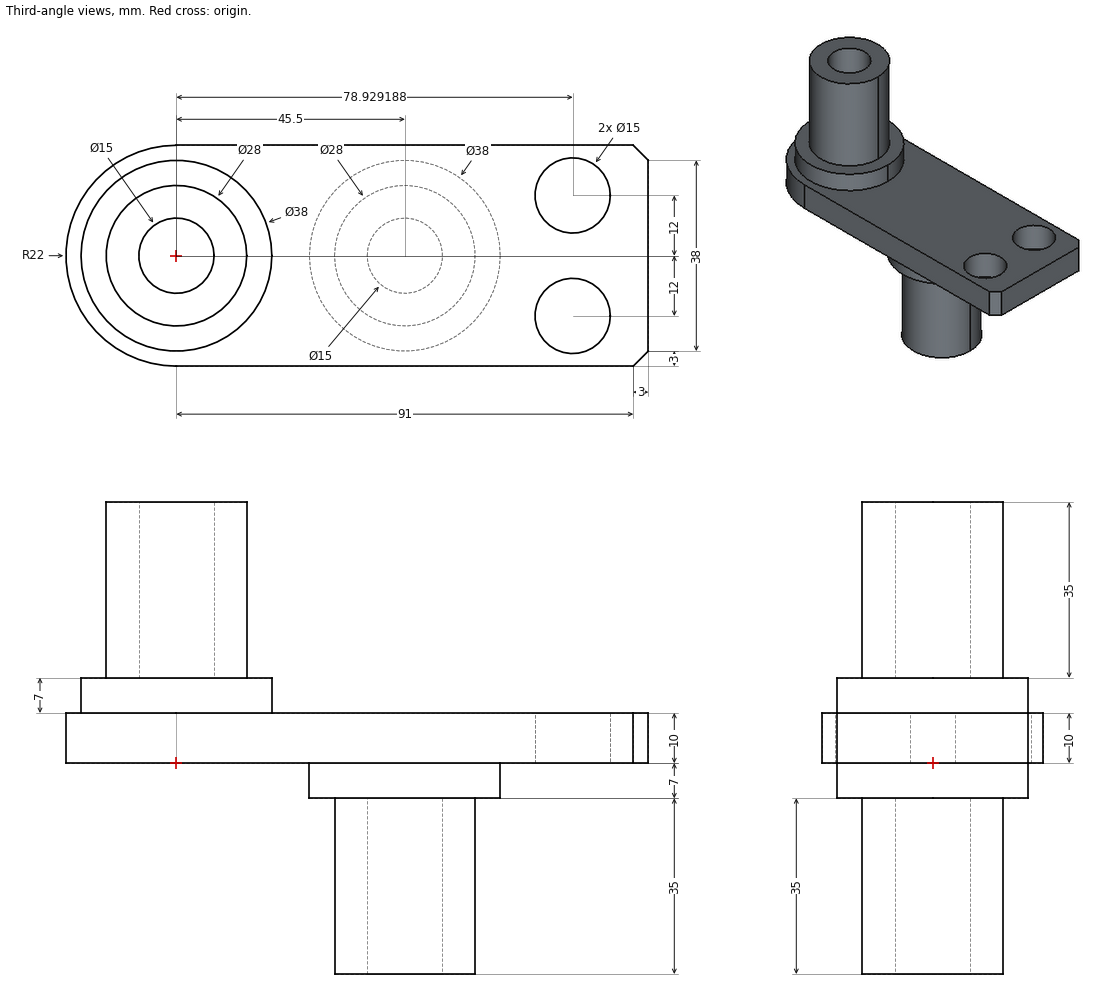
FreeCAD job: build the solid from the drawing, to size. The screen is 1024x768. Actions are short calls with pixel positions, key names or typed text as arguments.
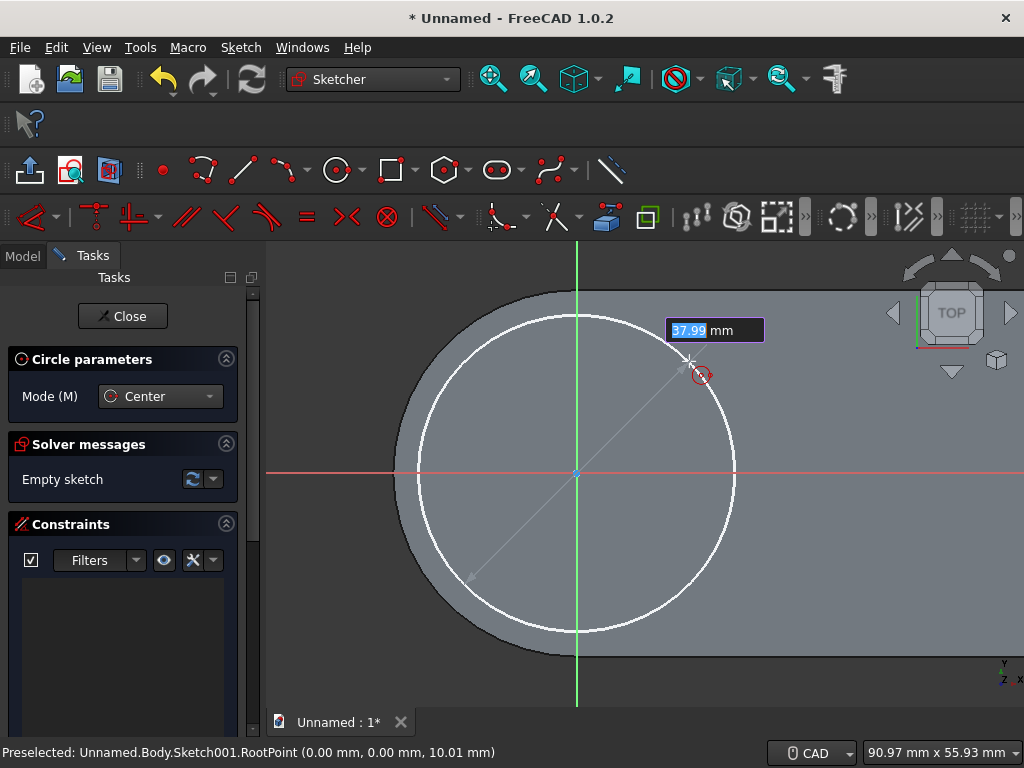
text(38)
key(Return)
key(Escape)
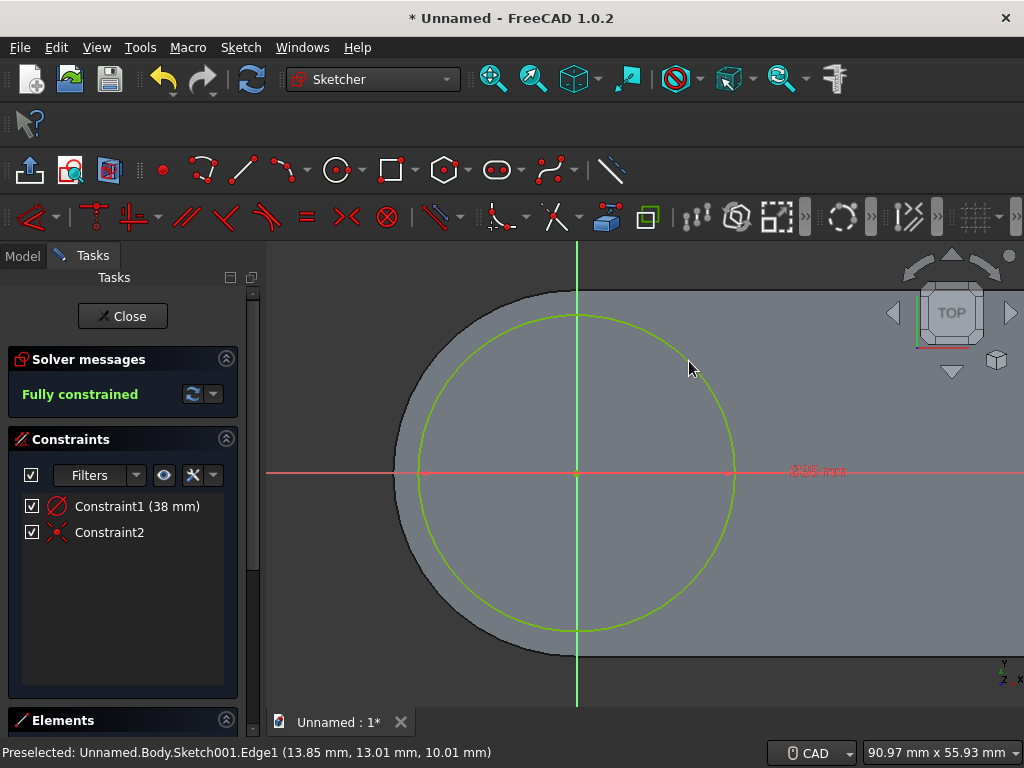
click(123, 316)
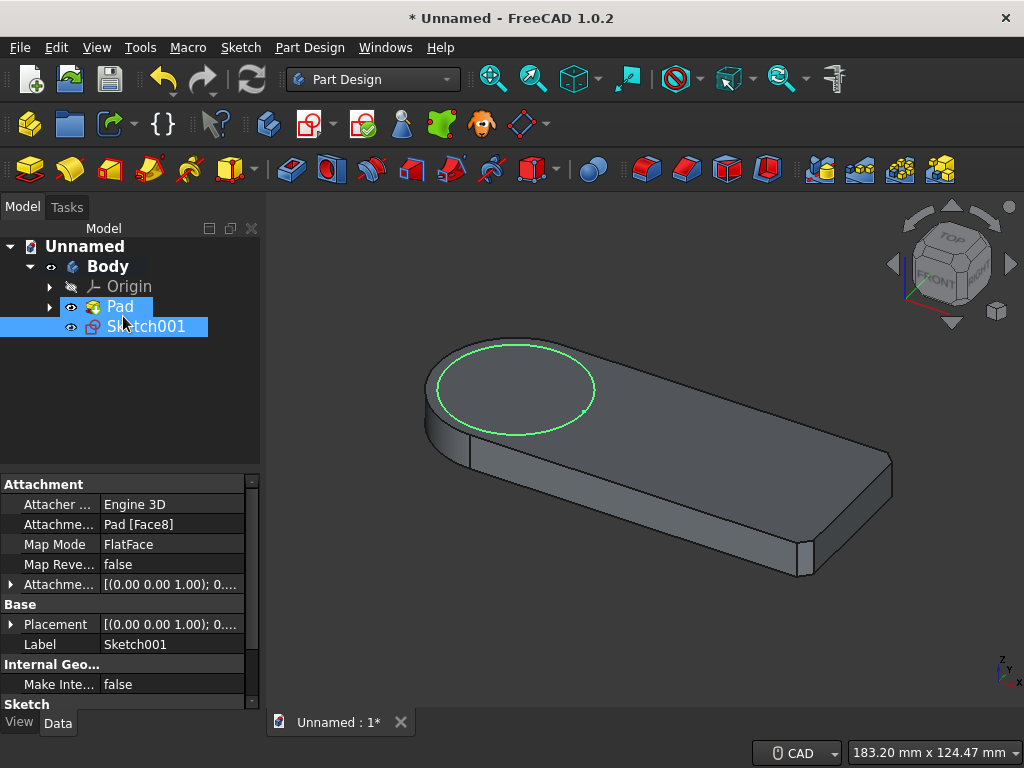
click(30, 170)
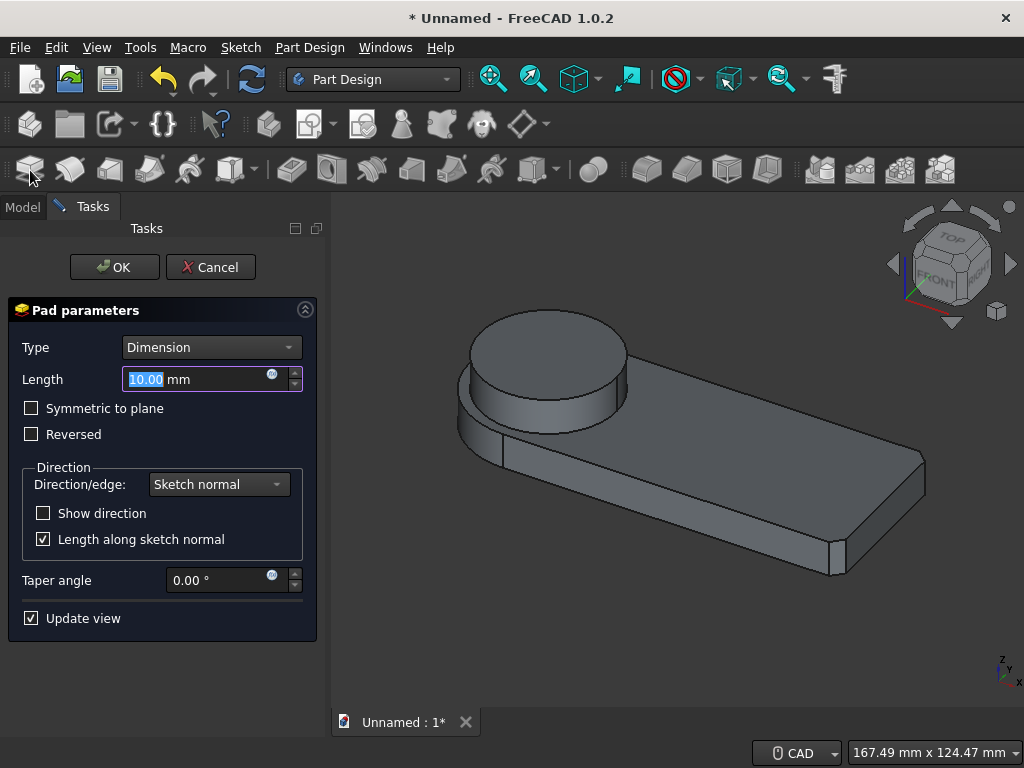
text(7)
key(Tab)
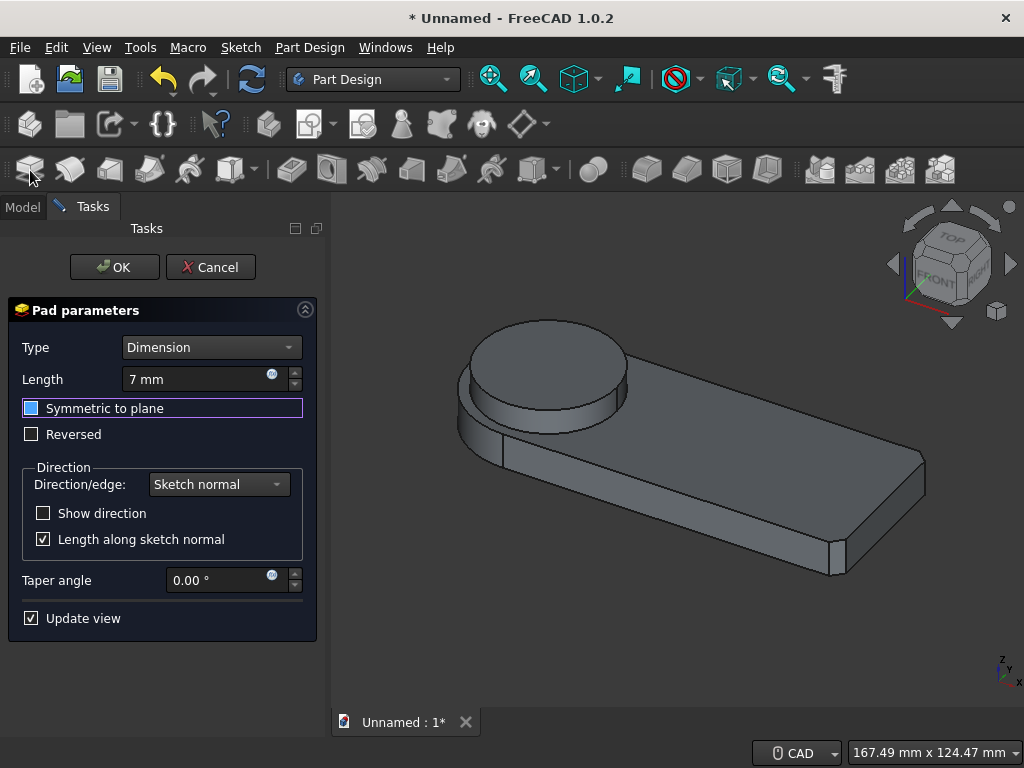
click(115, 267)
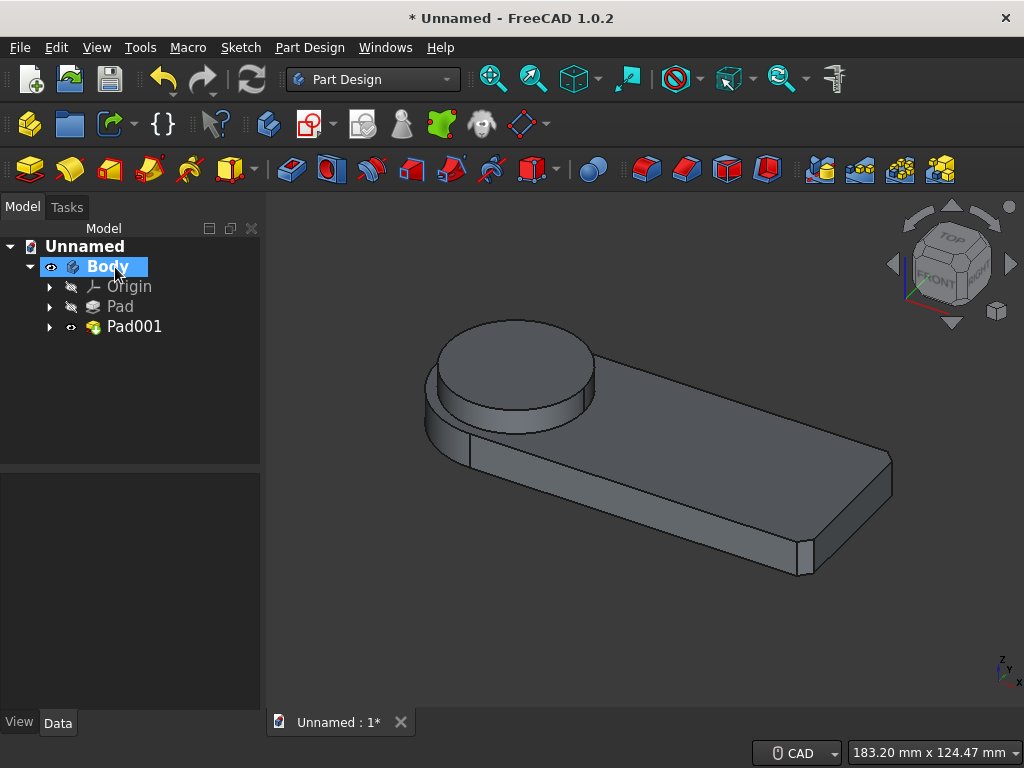
click(516, 364)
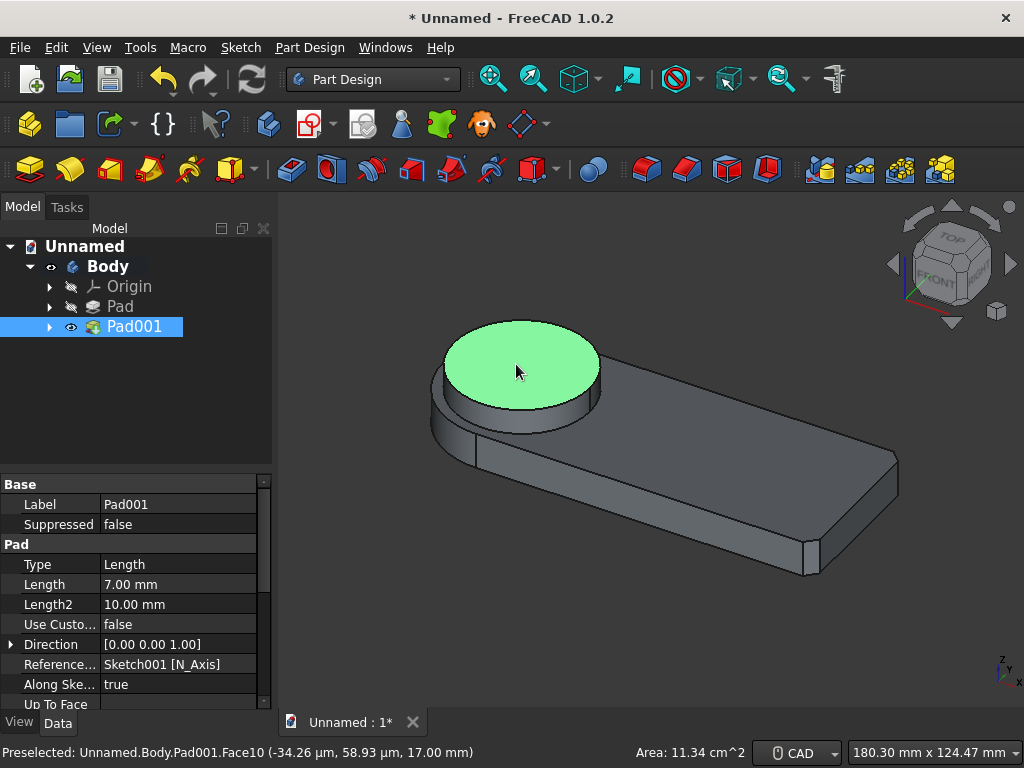
click(310, 124)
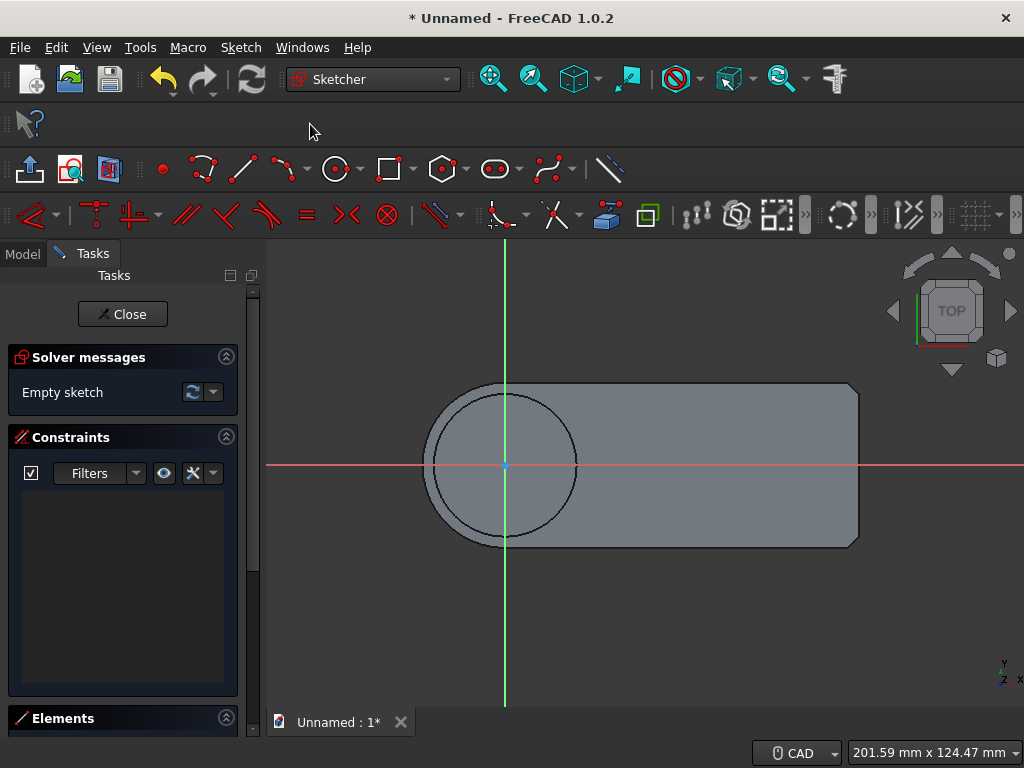
scroll(464, 461, up, 5)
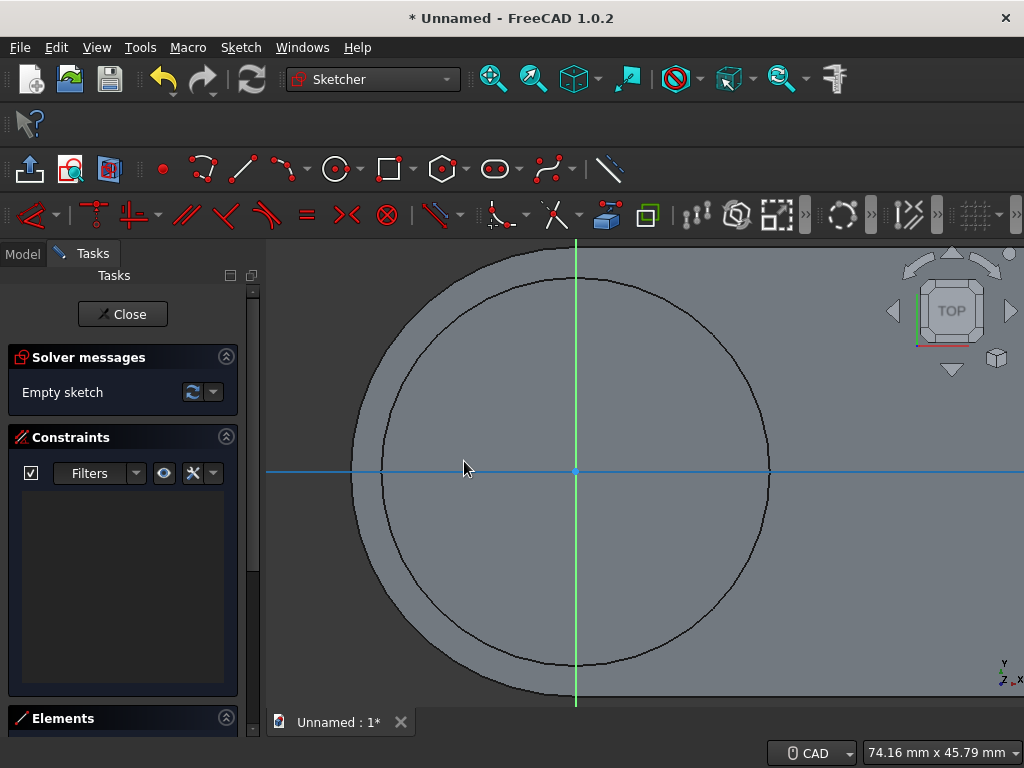
click(336, 170)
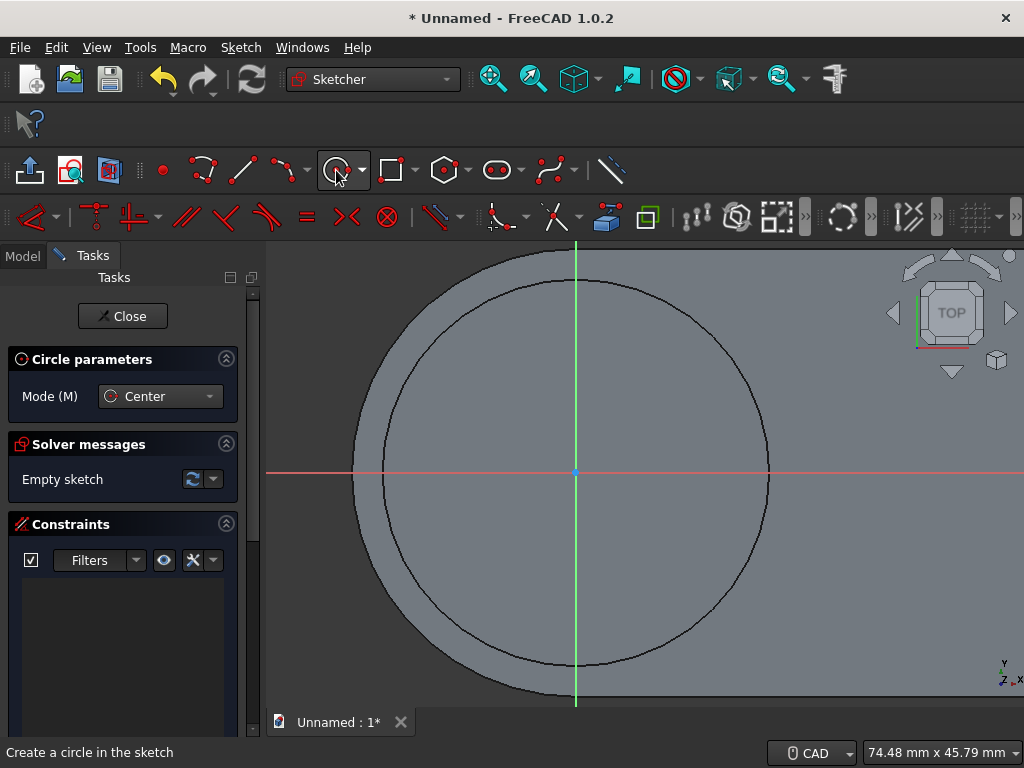
click(576, 473)
move(677, 372)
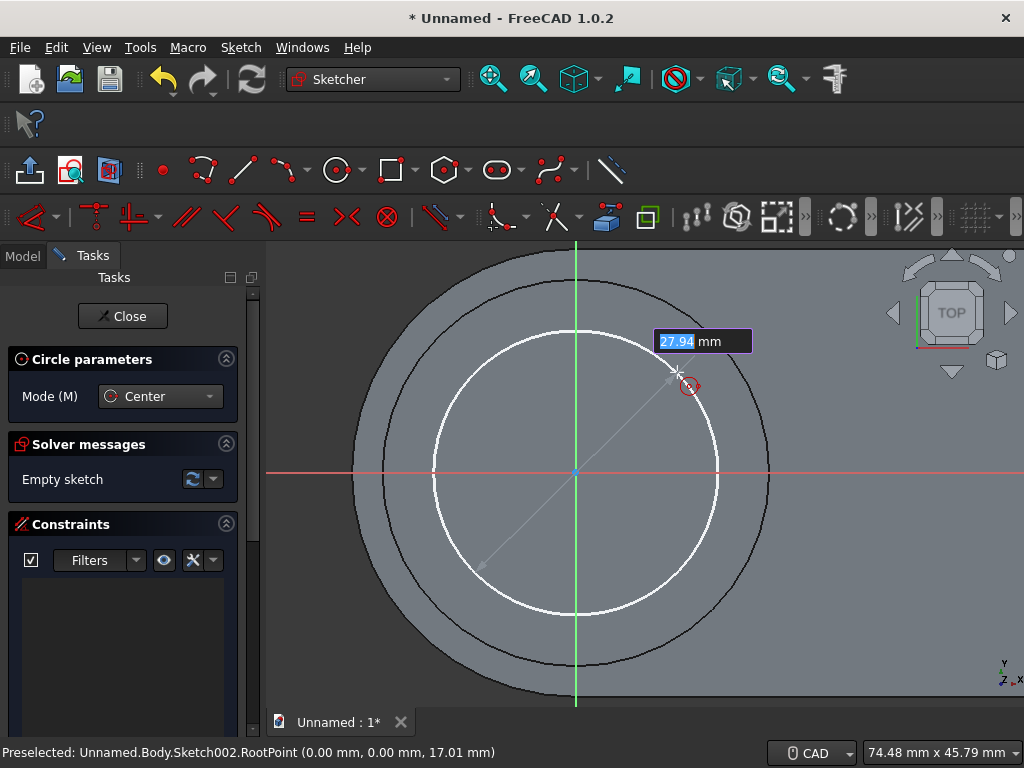
text(28)
key(Return)
key(Escape)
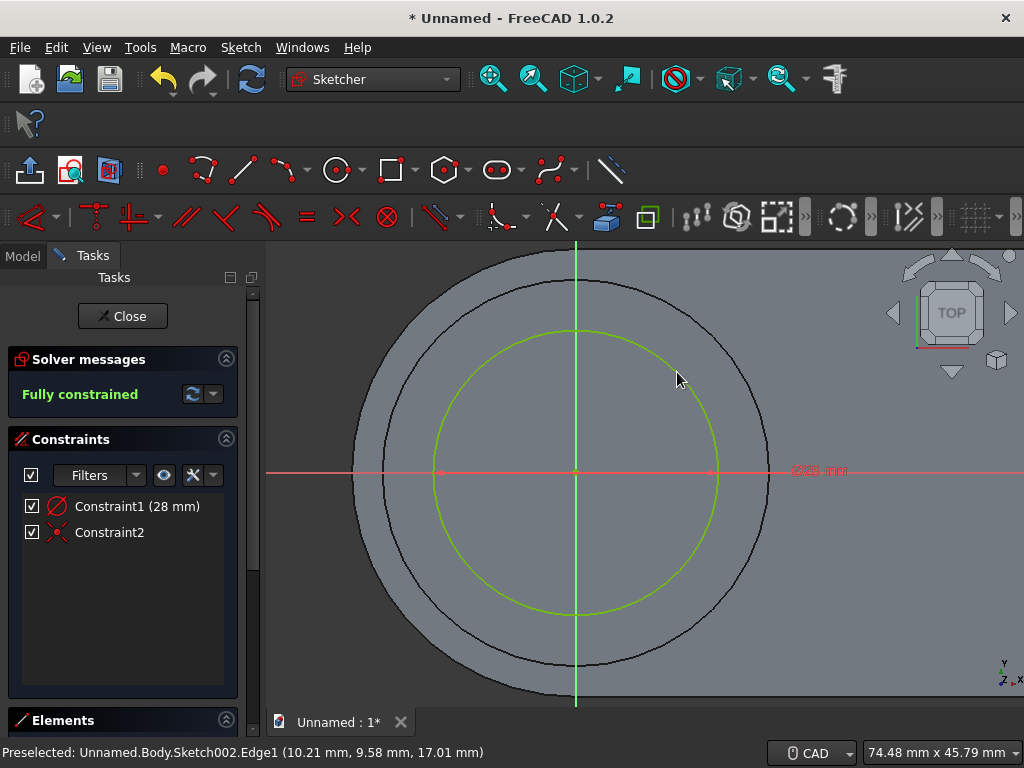
click(123, 316)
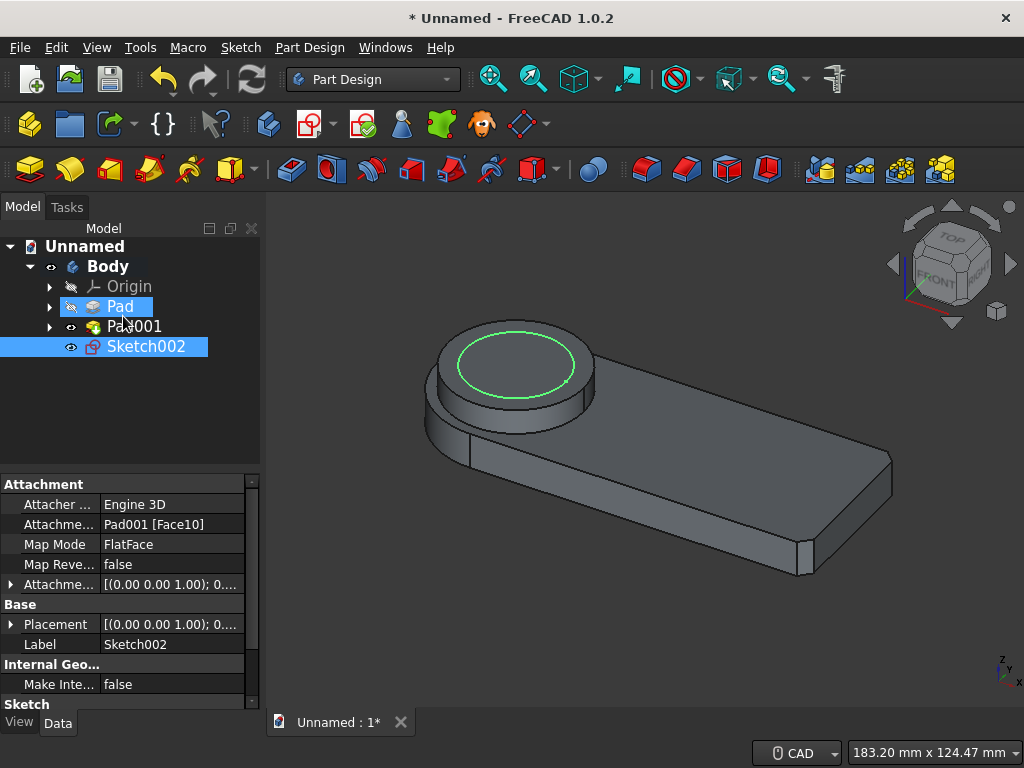
click(30, 170)